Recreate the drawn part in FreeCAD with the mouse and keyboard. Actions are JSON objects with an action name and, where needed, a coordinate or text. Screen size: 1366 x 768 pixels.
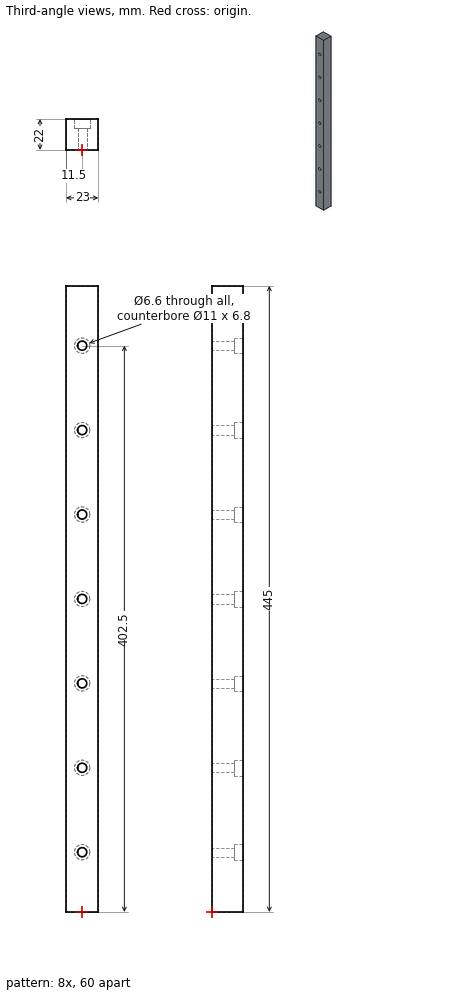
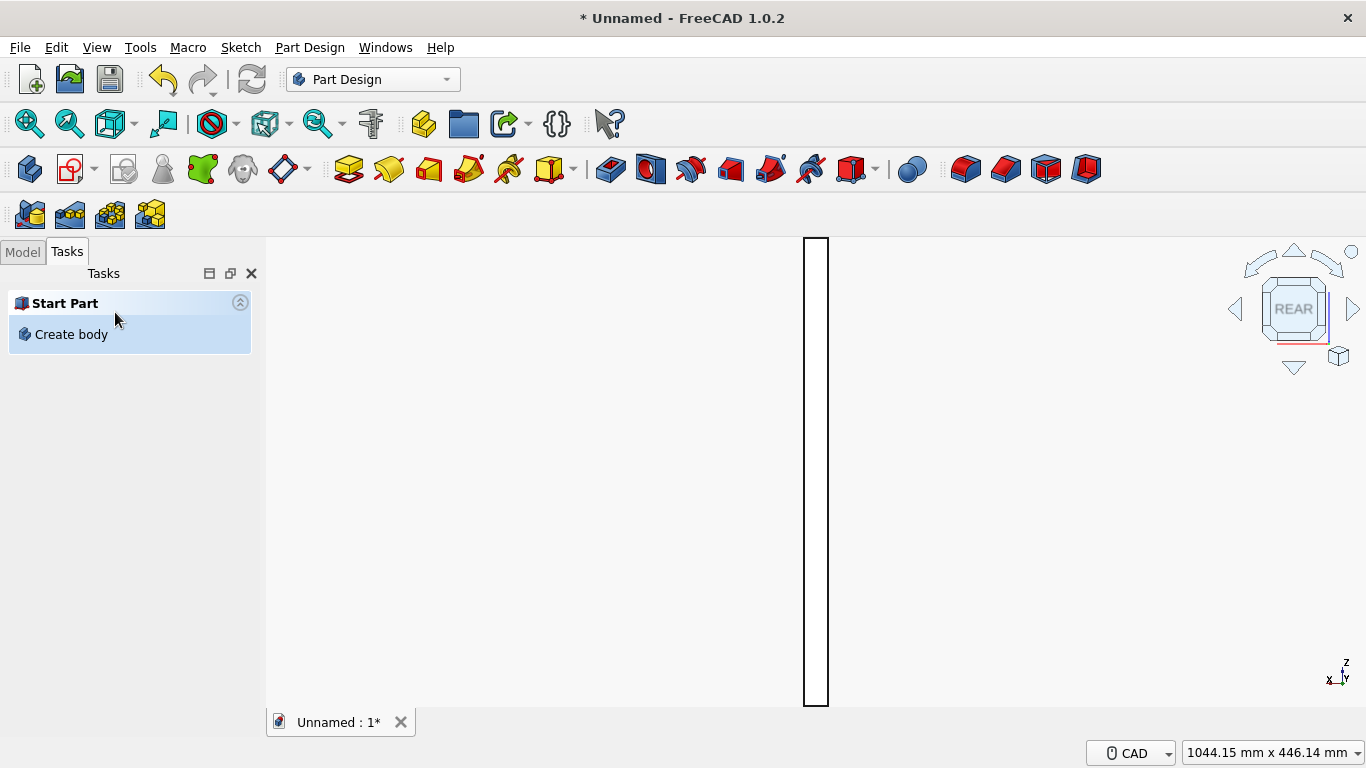
{"action": "left_click", "coordinate": [816, 270]}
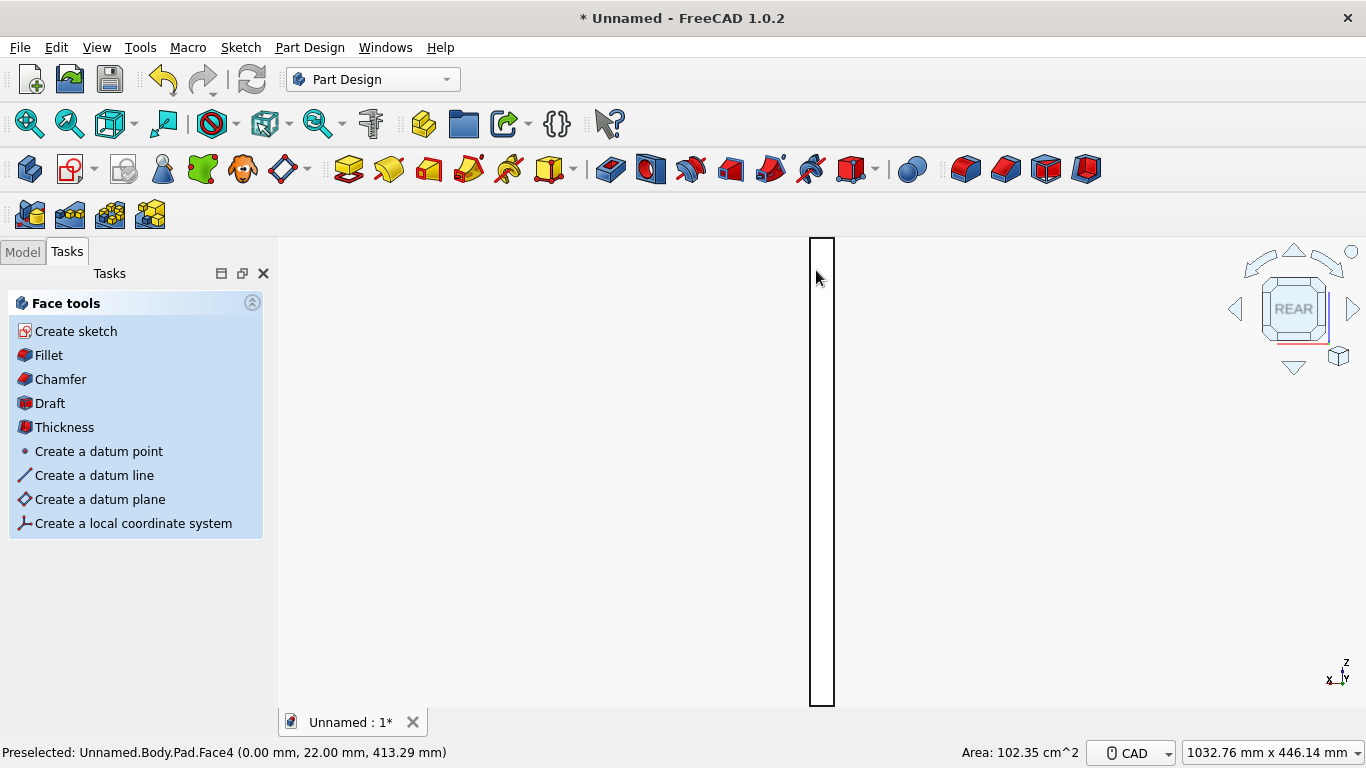
{"action": "left_click", "coordinate": [70, 170]}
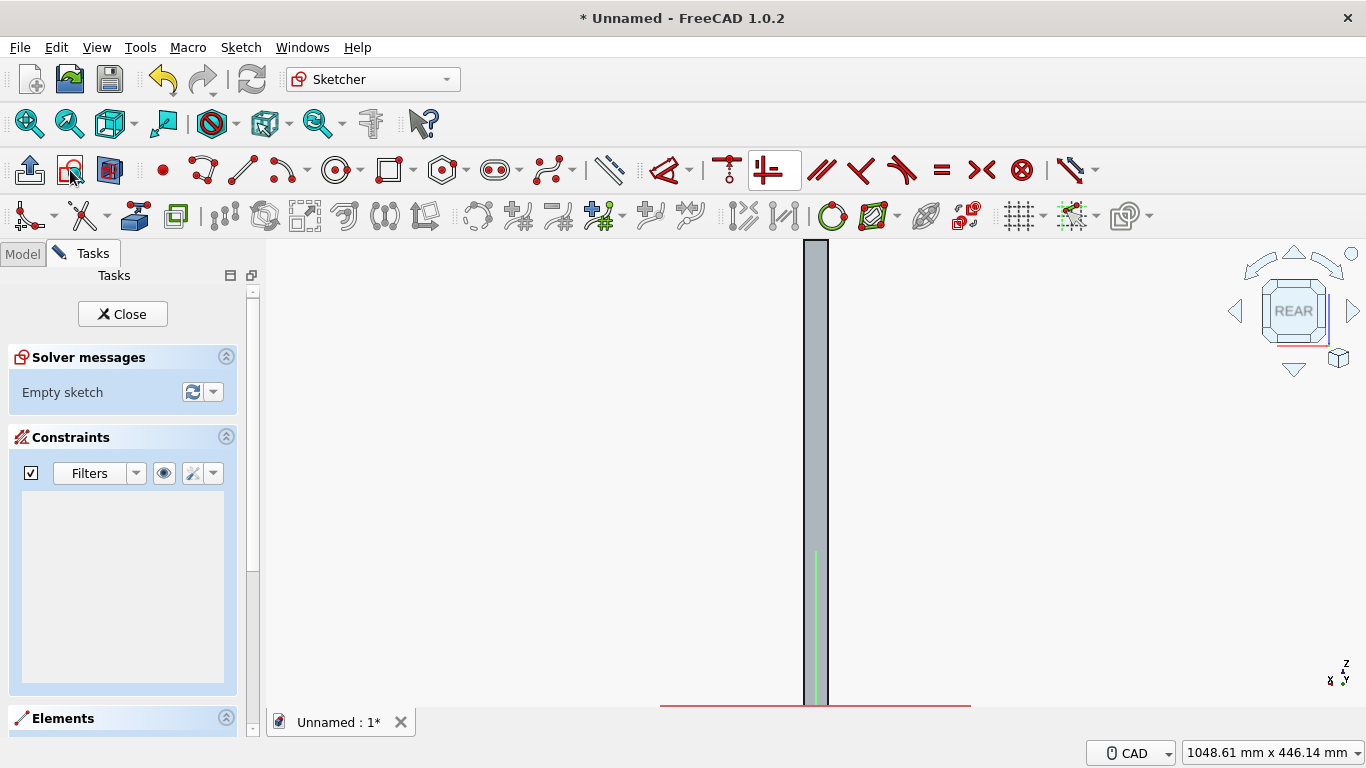
{"action": "scroll", "coordinate": [820, 274], "scroll_direction": "up", "scroll_amount": 15}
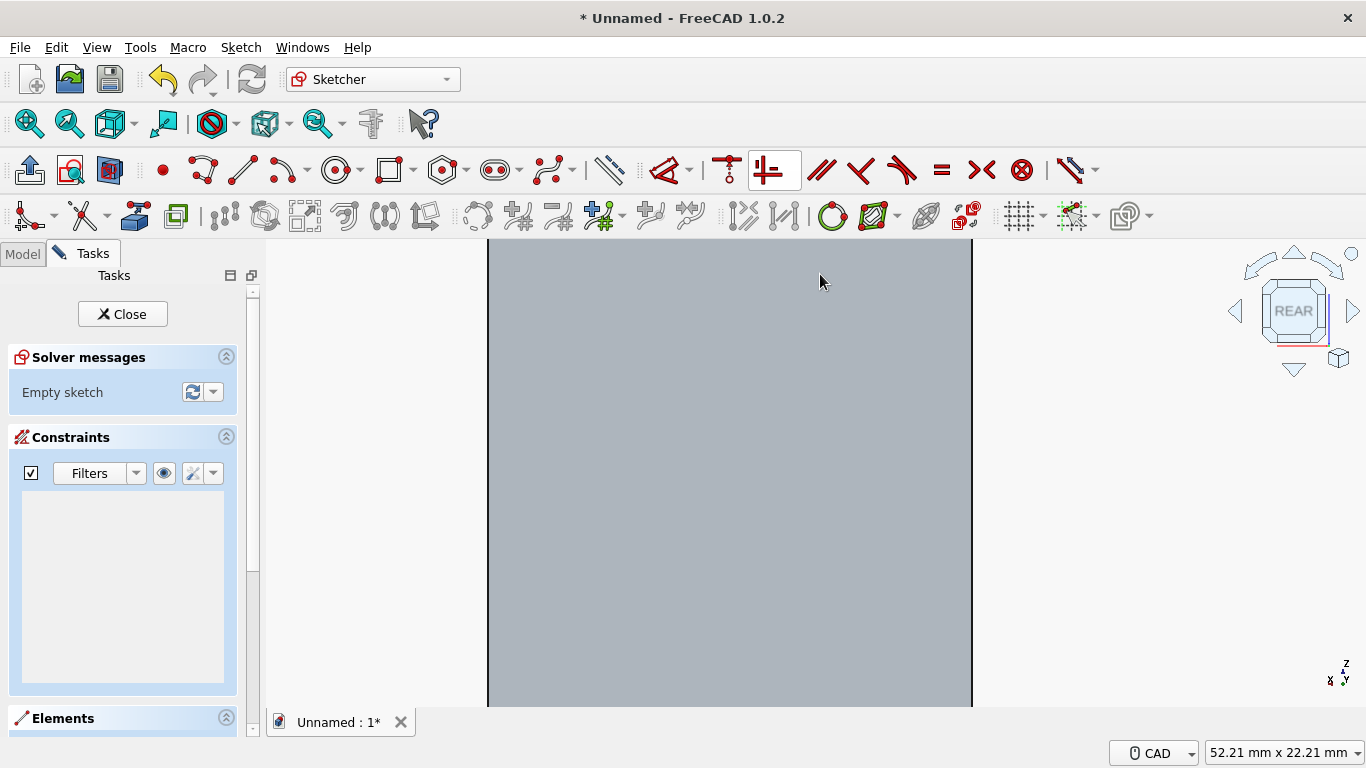
{"action": "scroll", "coordinate": [716, 480], "scroll_direction": "up", "scroll_amount": 4}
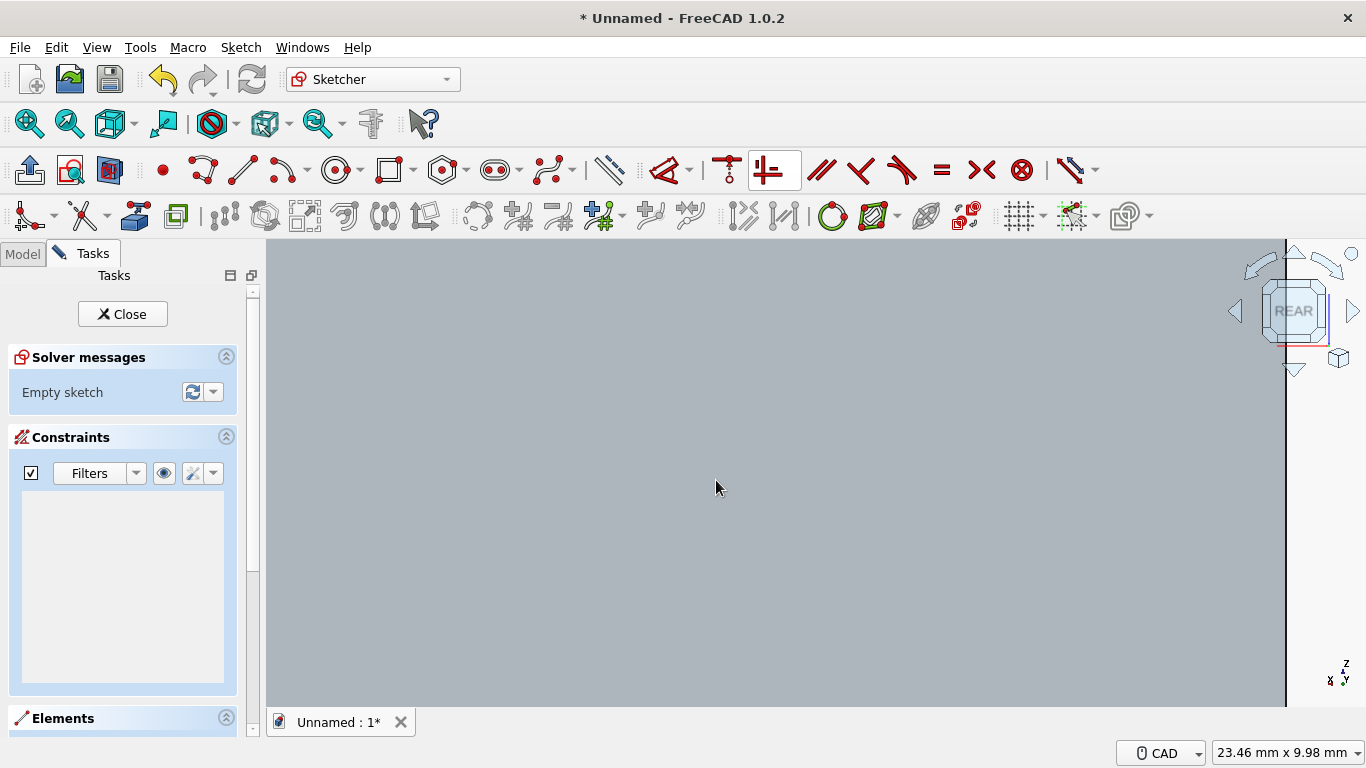
{"action": "key", "text": "g c"}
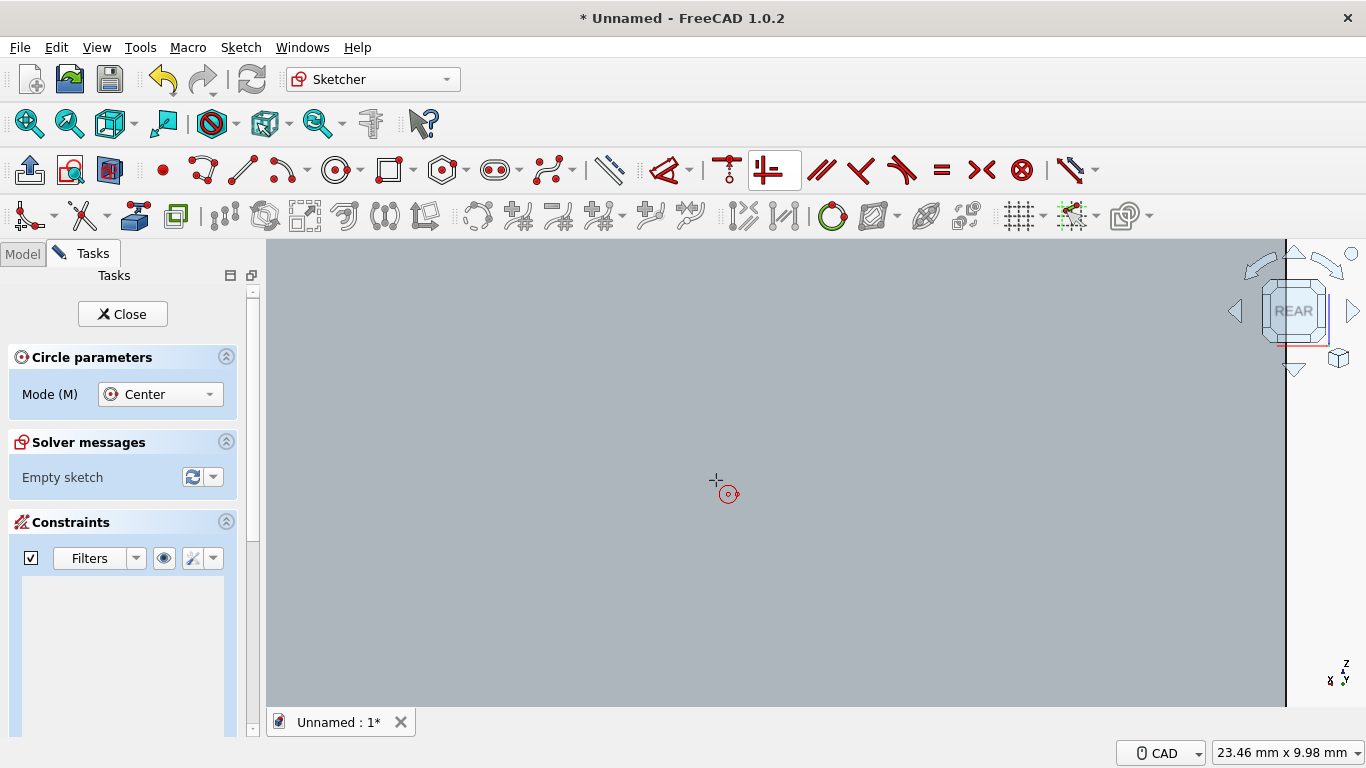
{"action": "left_click", "coordinate": [747, 473]}
{"action": "left_click", "coordinate": [856, 363]}
{"action": "key", "text": "Escape"}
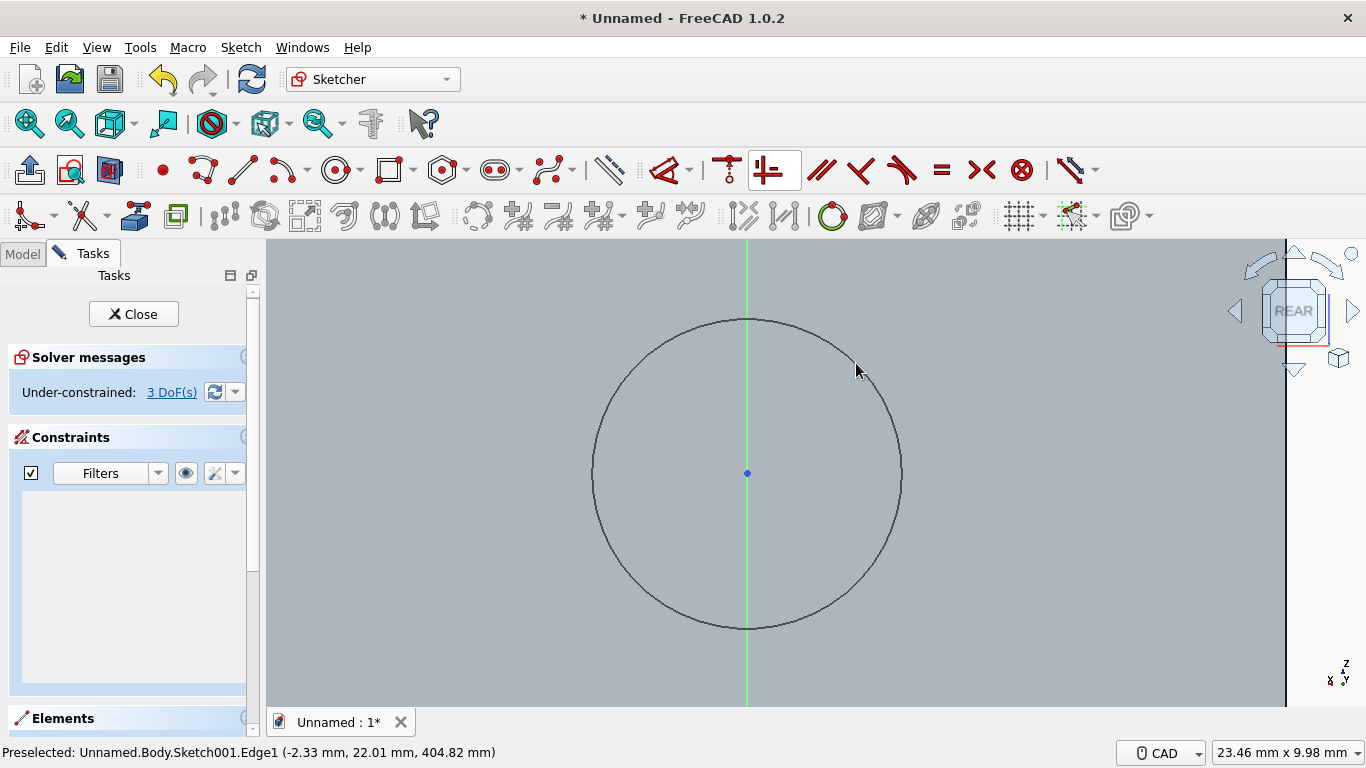
{"action": "left_click", "coordinate": [747, 474]}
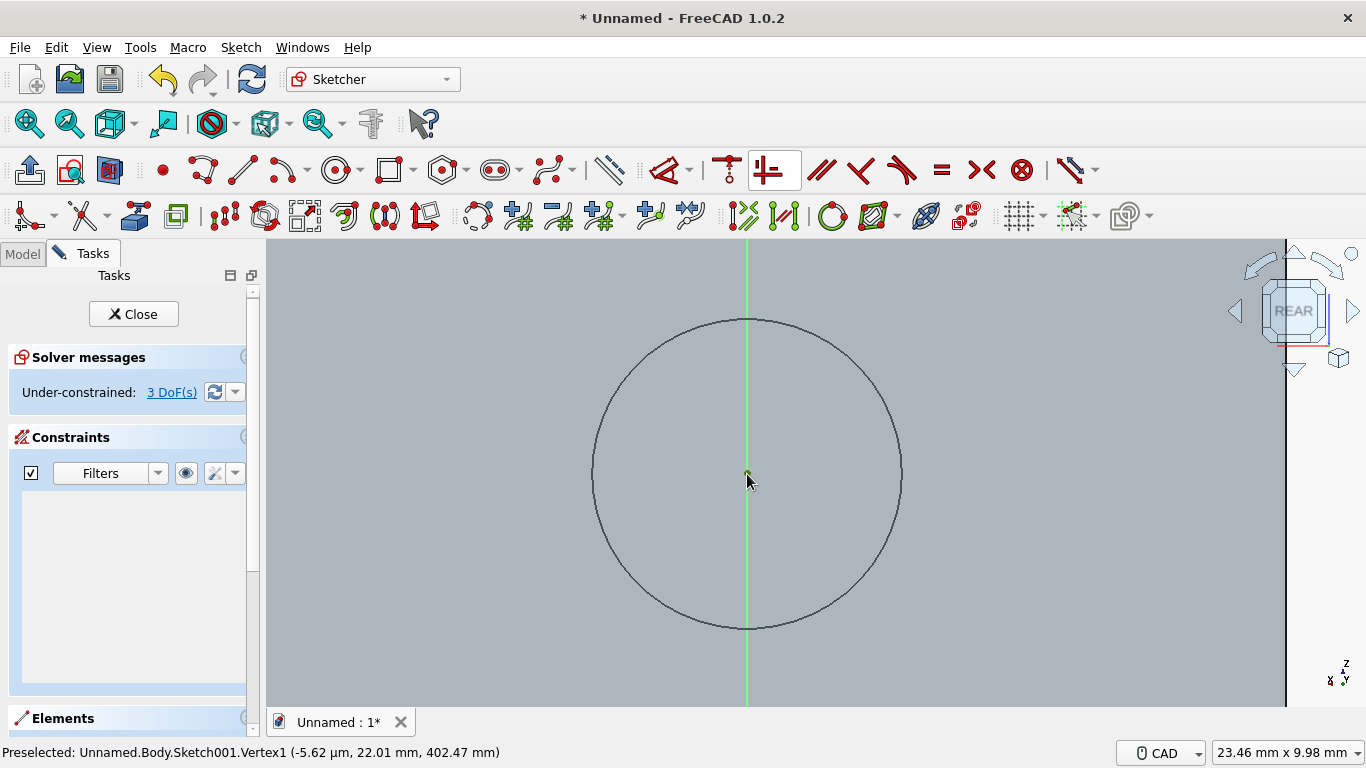
{"action": "left_click", "coordinate": [747, 591]}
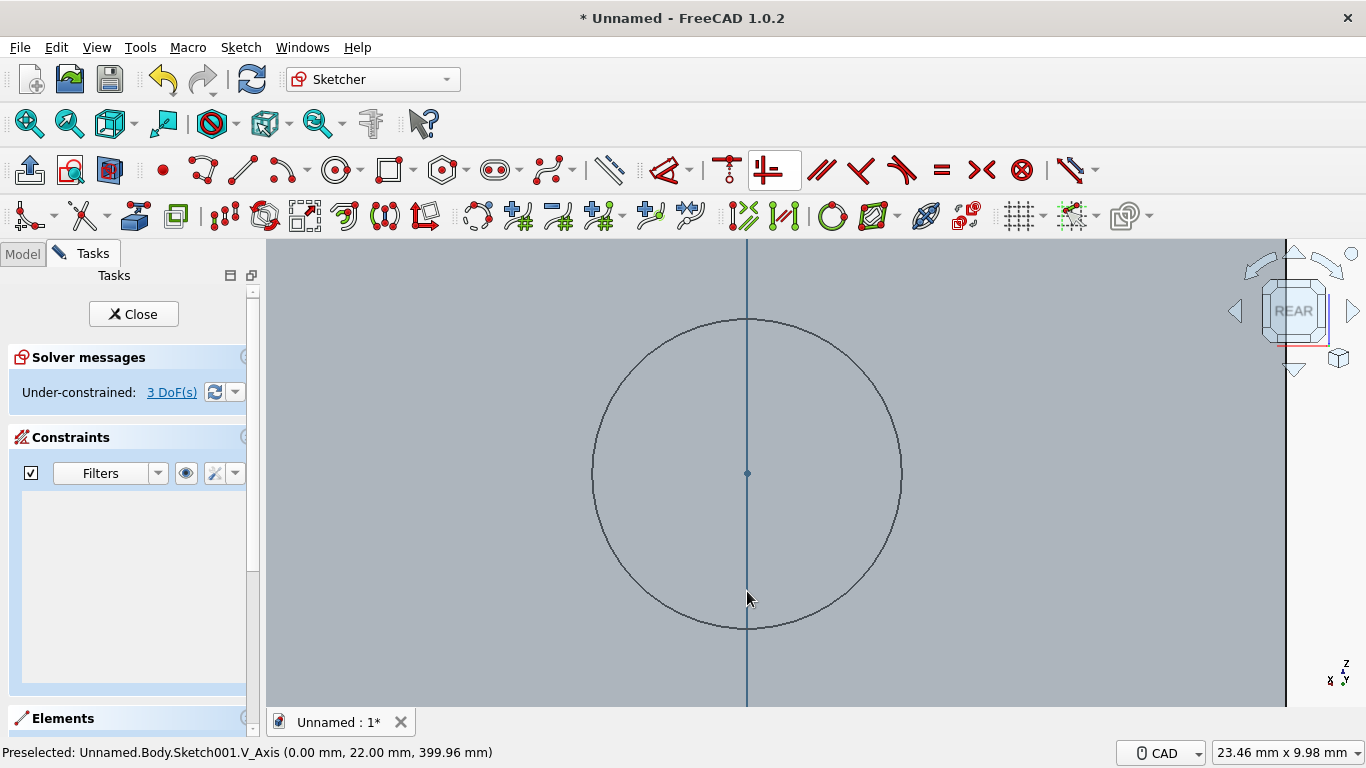
{"action": "key", "text": "c"}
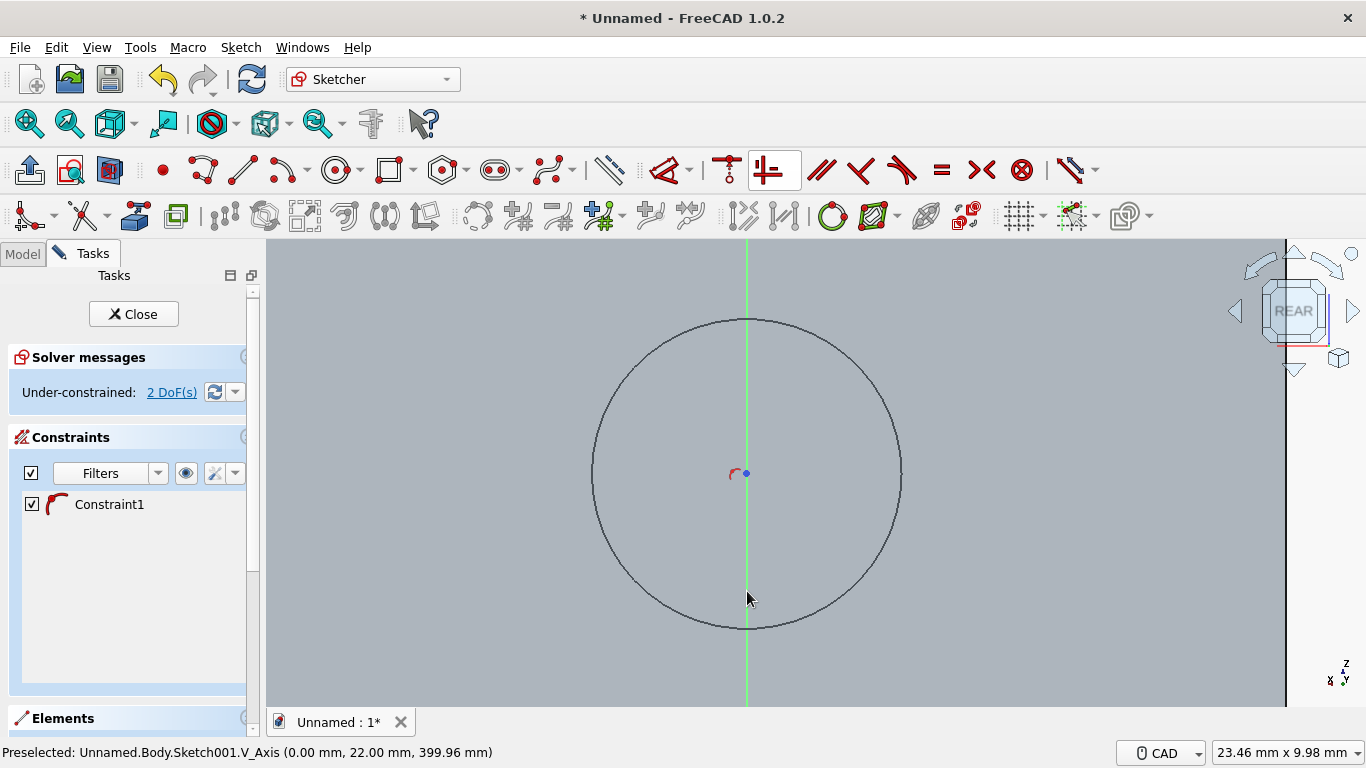
{"action": "key", "text": "d"}